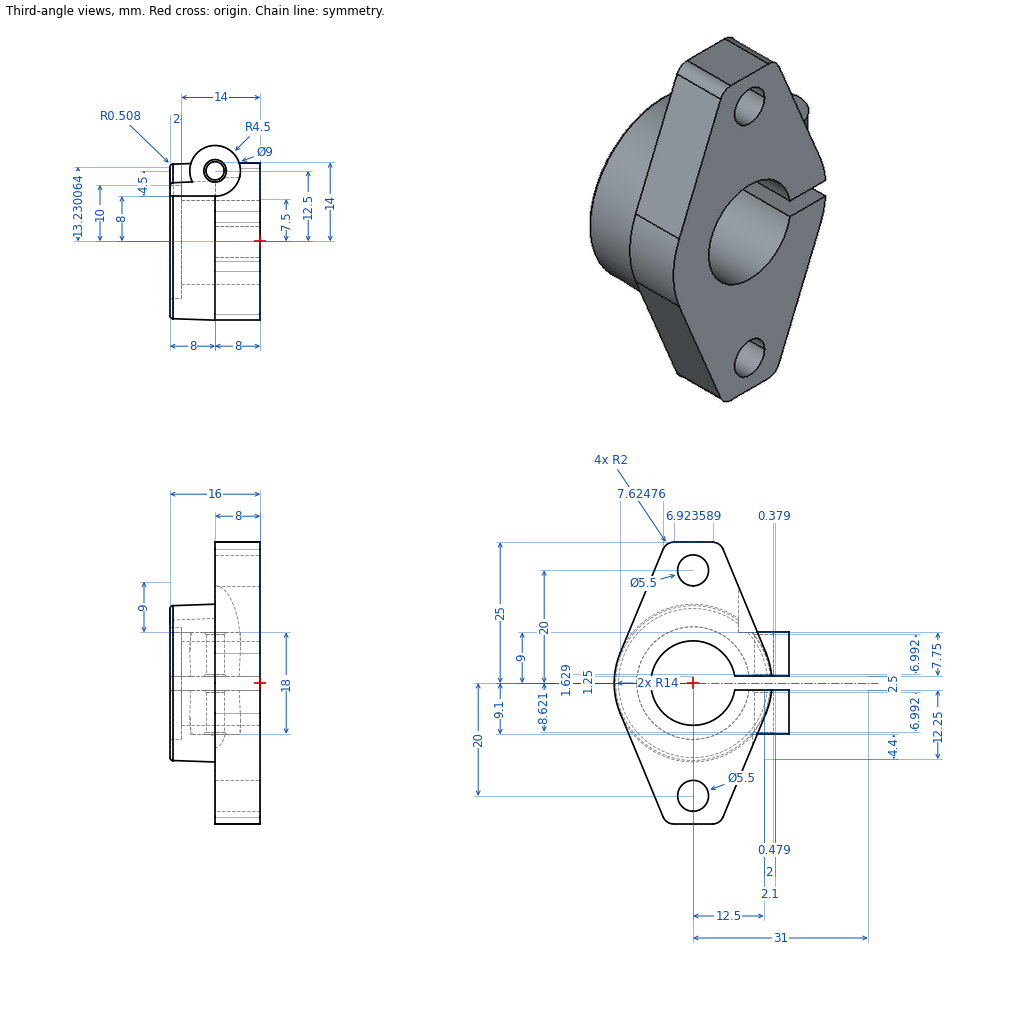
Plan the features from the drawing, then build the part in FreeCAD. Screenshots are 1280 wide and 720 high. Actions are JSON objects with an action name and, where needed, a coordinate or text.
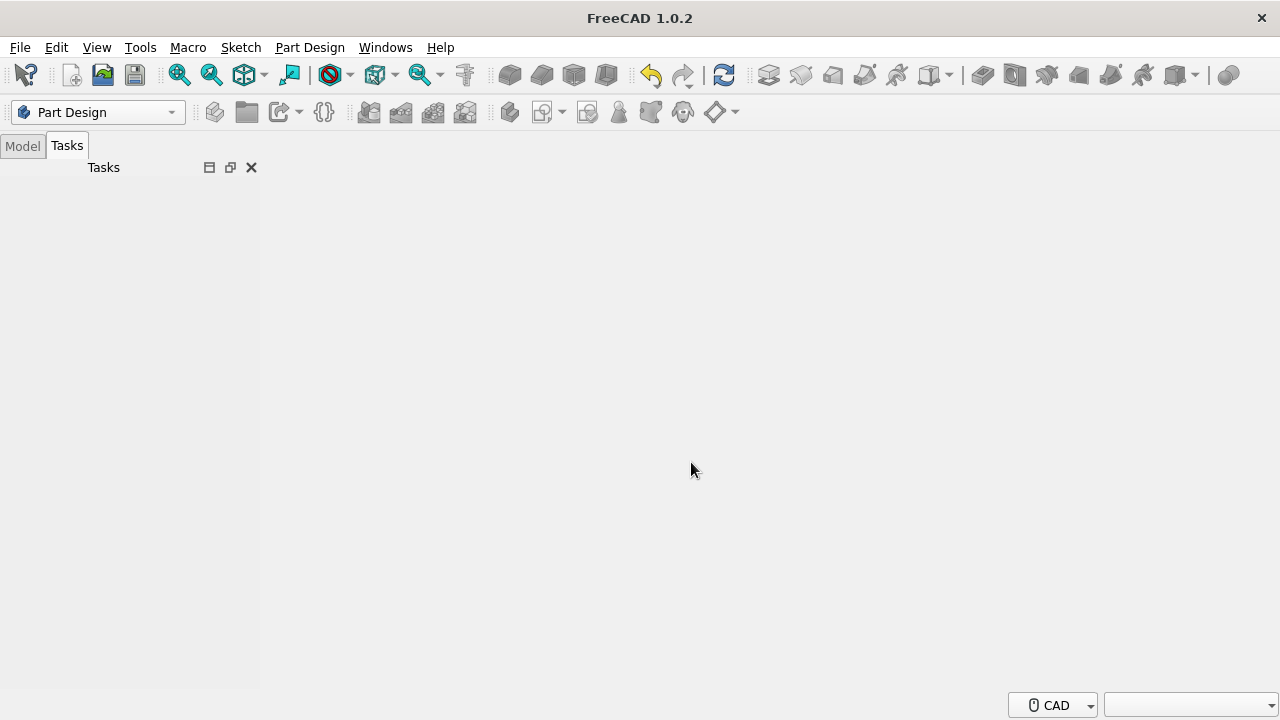
{"action": "key", "text": "ctrl+n"}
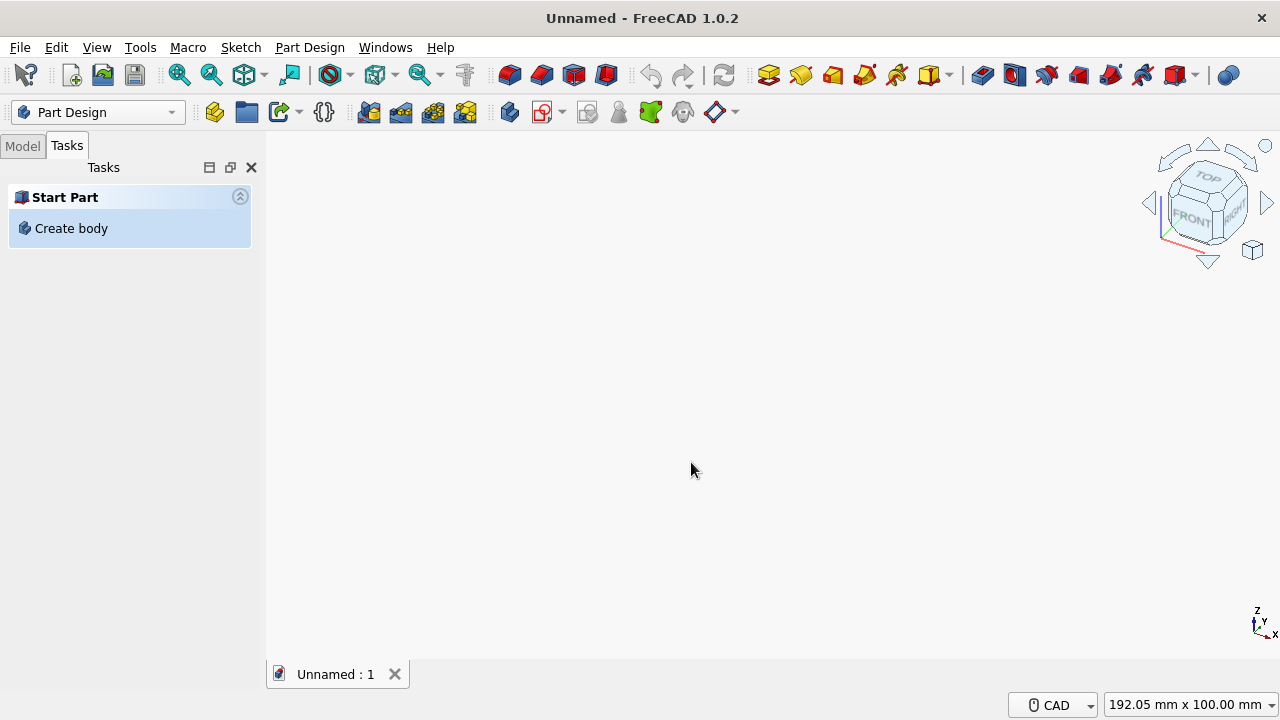
{"action": "left_click", "coordinate": [542, 112]}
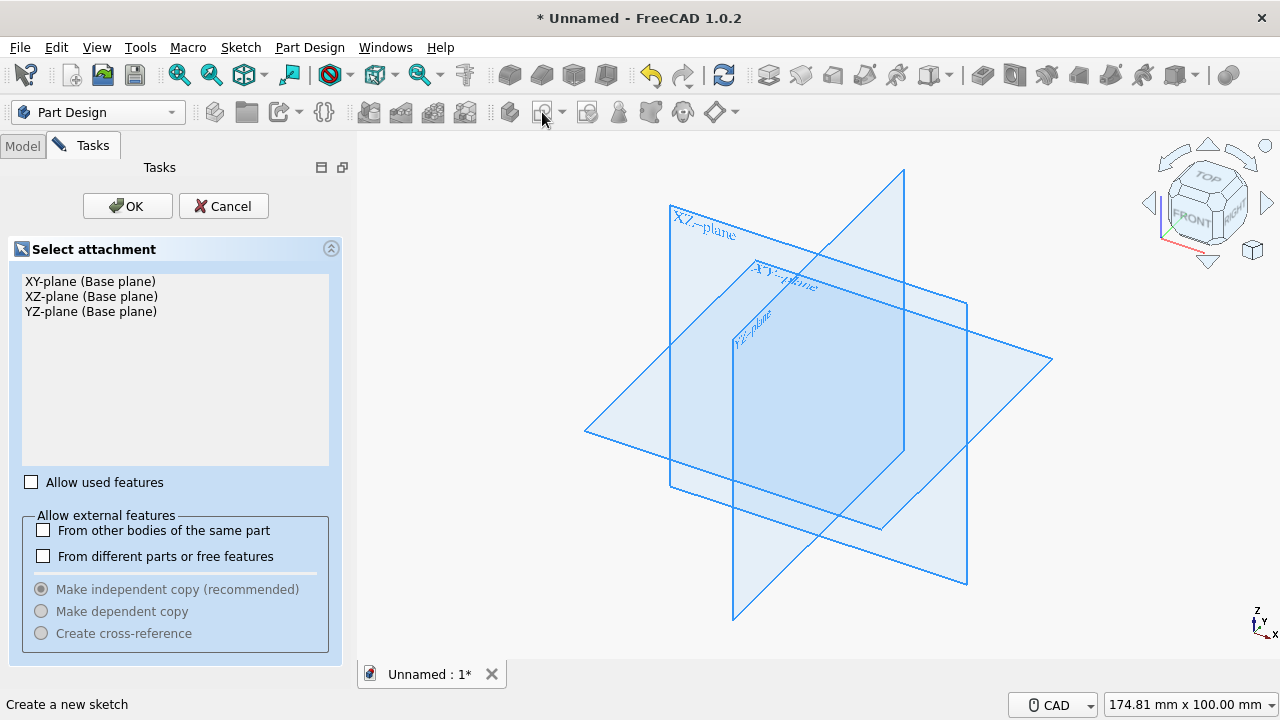
{"action": "left_click", "coordinate": [82, 312]}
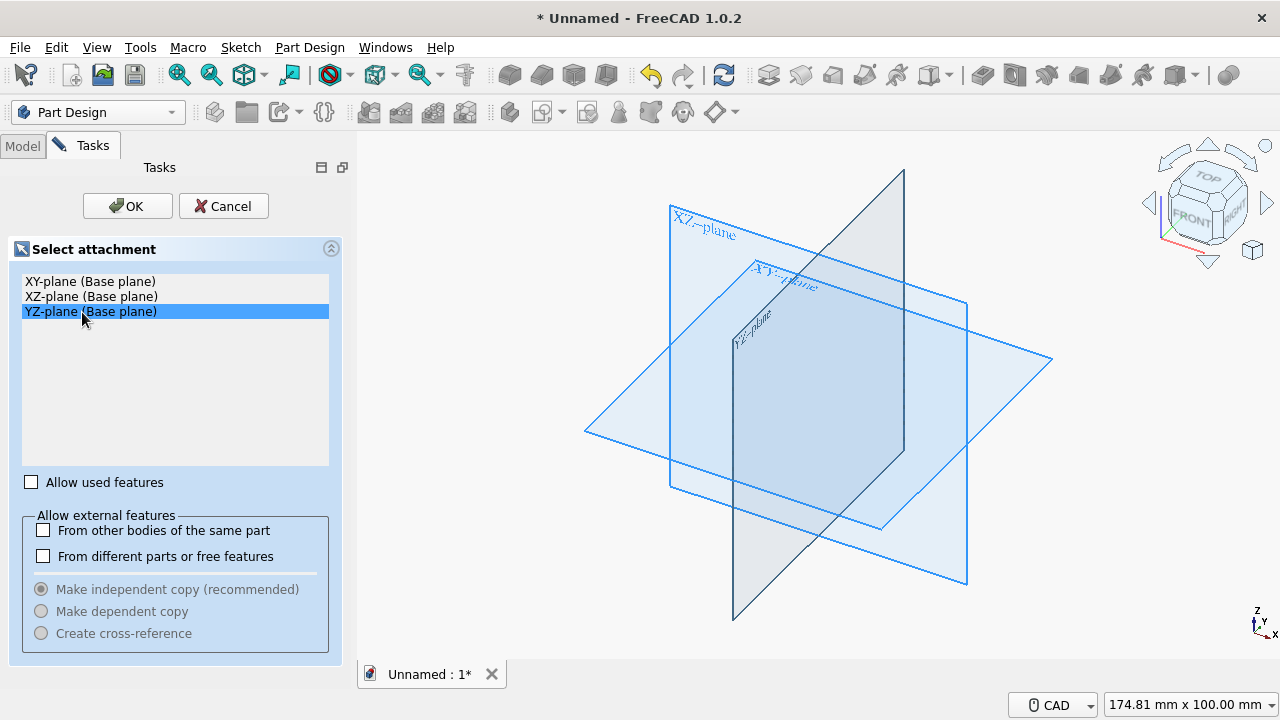
{"action": "left_click", "coordinate": [128, 206]}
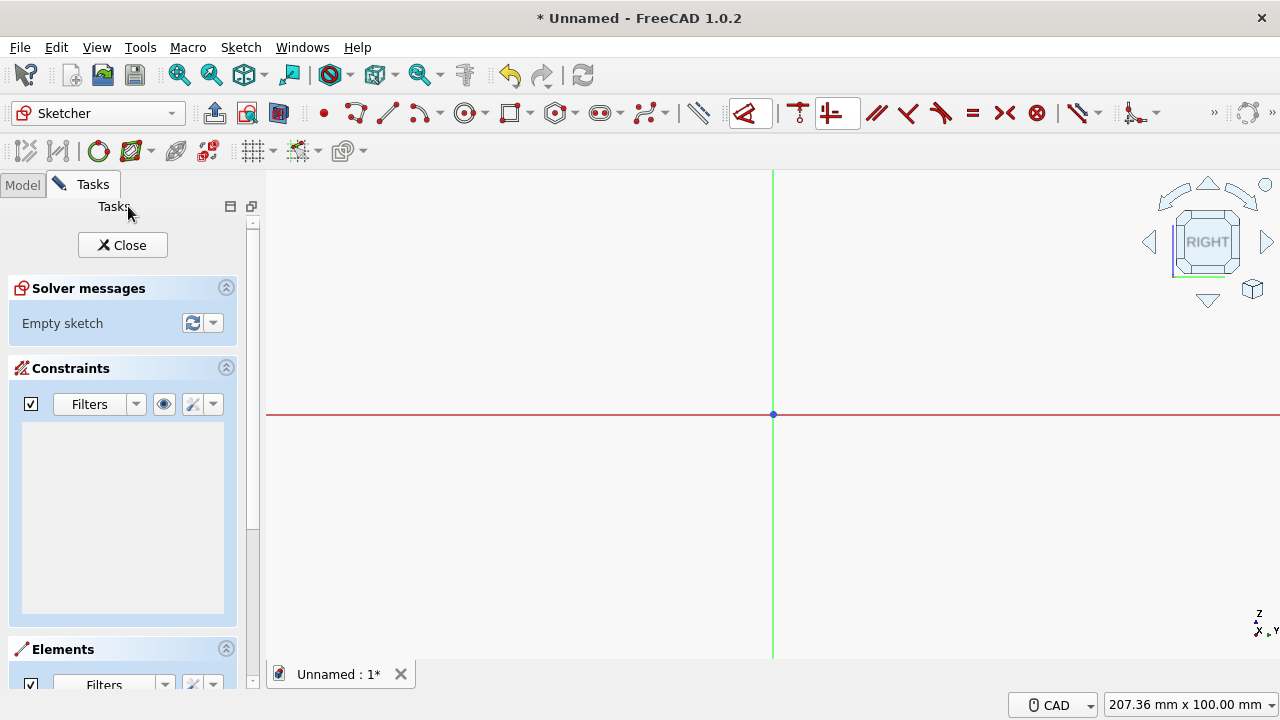
{"action": "key", "text": "g l"}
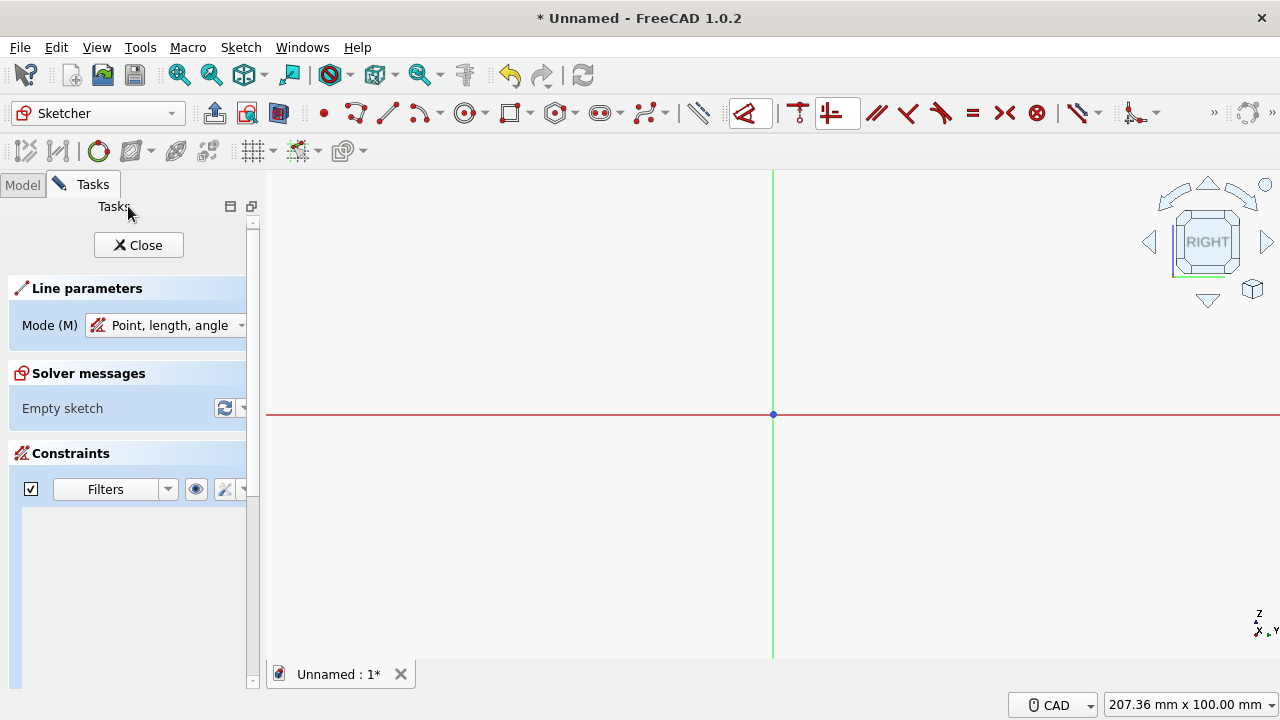
{"action": "left_click", "coordinate": [790, 292]}
{"action": "left_click", "coordinate": [756, 292]}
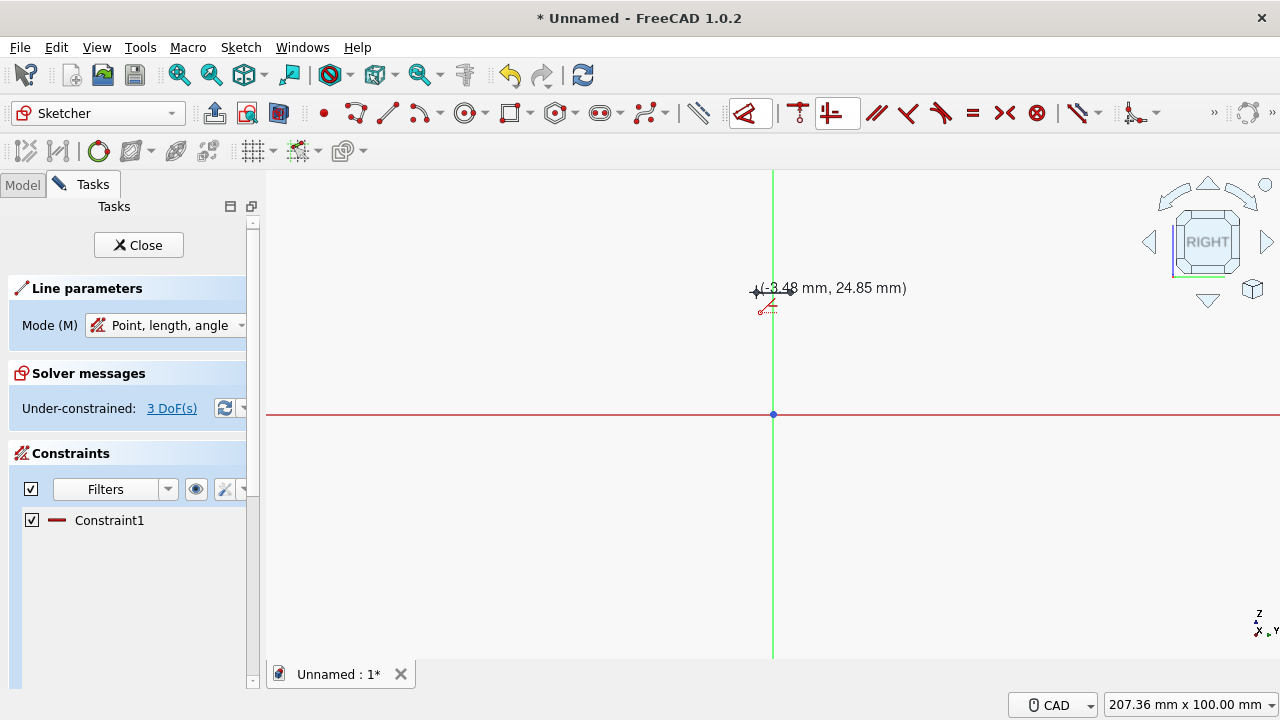
{"action": "scroll", "coordinate": [747, 298], "scroll_direction": "up", "scroll_amount": 2}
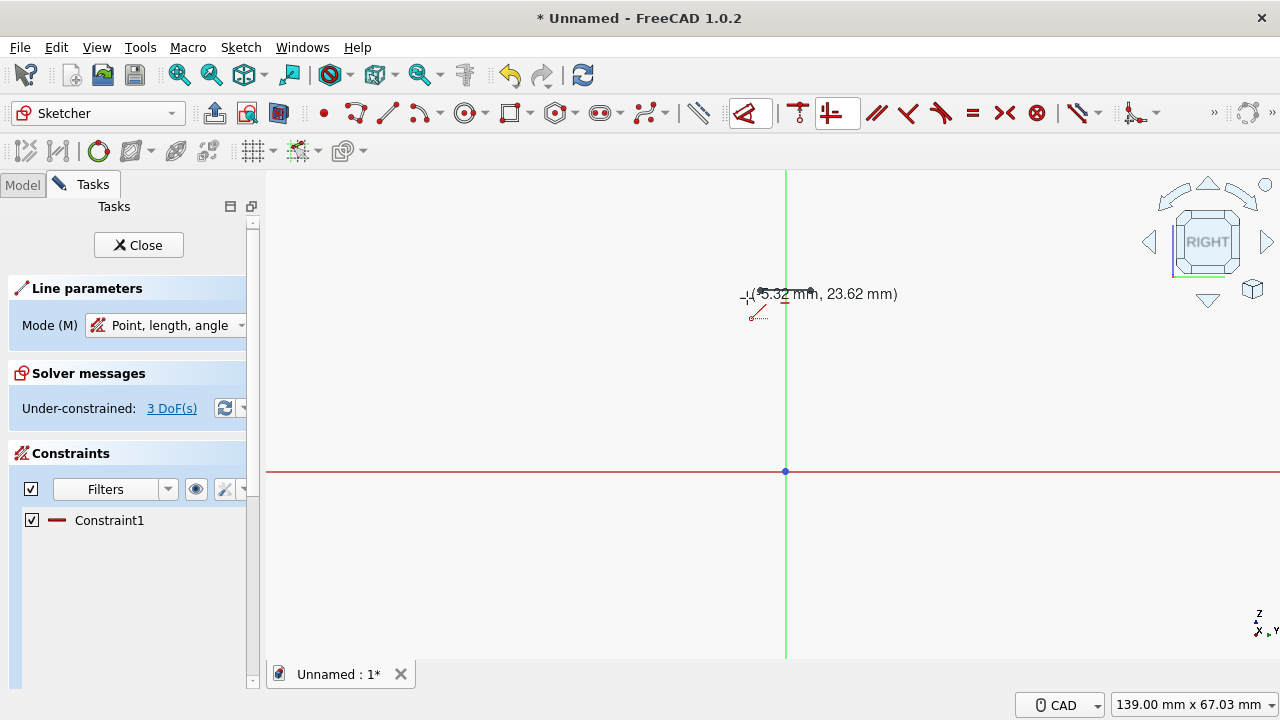
{"action": "left_click", "coordinate": [747, 298]}
{"action": "left_click", "coordinate": [691, 433]}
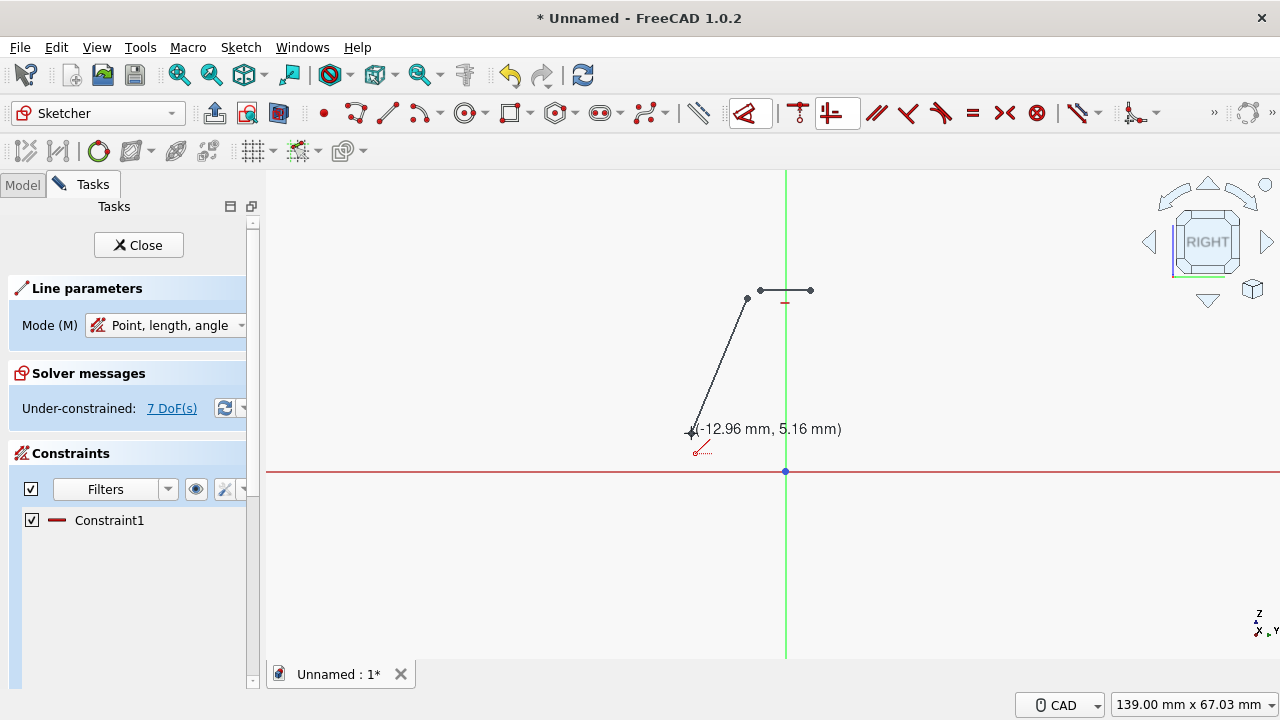
{"action": "left_click", "coordinate": [691, 511]}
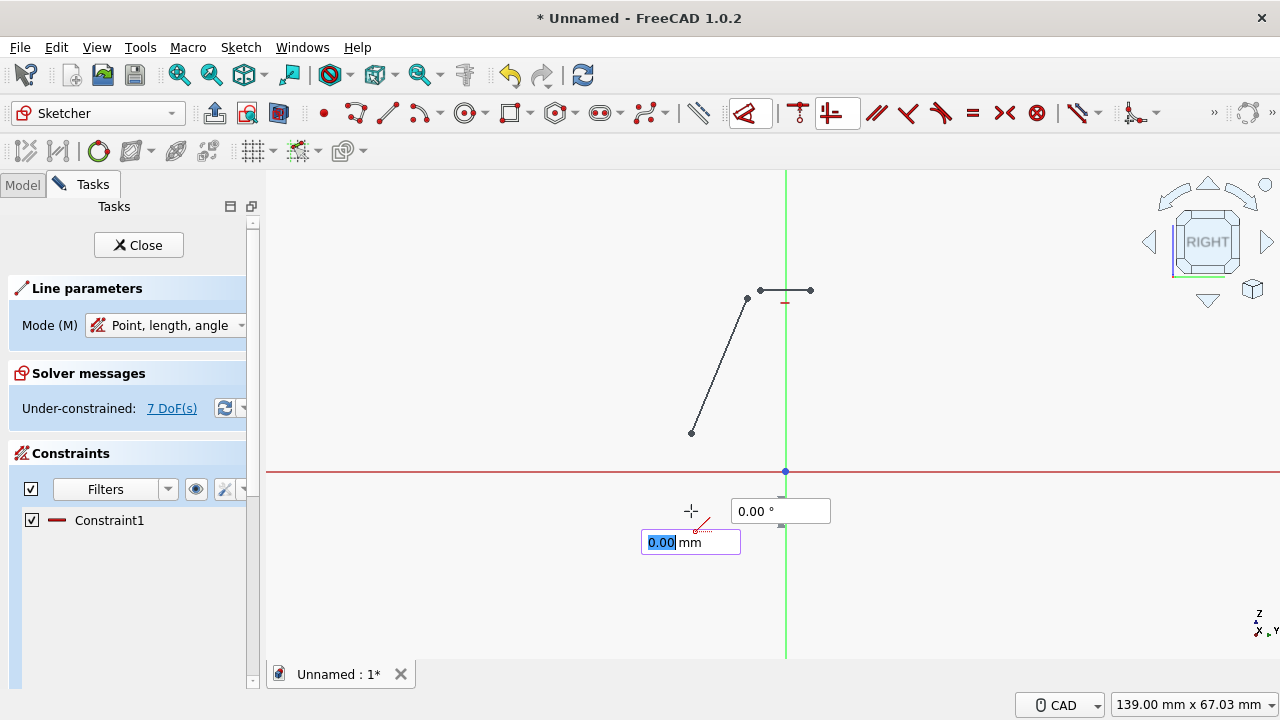
{"action": "scroll", "coordinate": [338, 198], "scroll_direction": "down", "scroll_amount": 1}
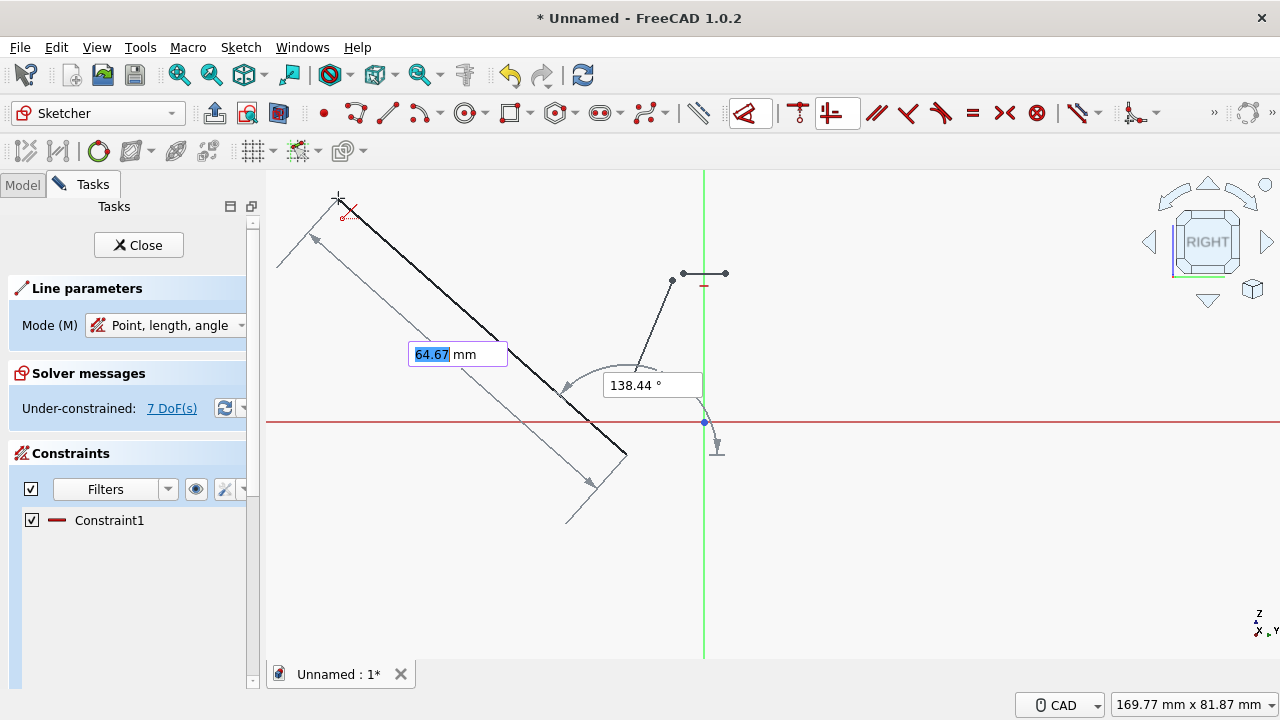
{"action": "left_click", "coordinate": [673, 564]}